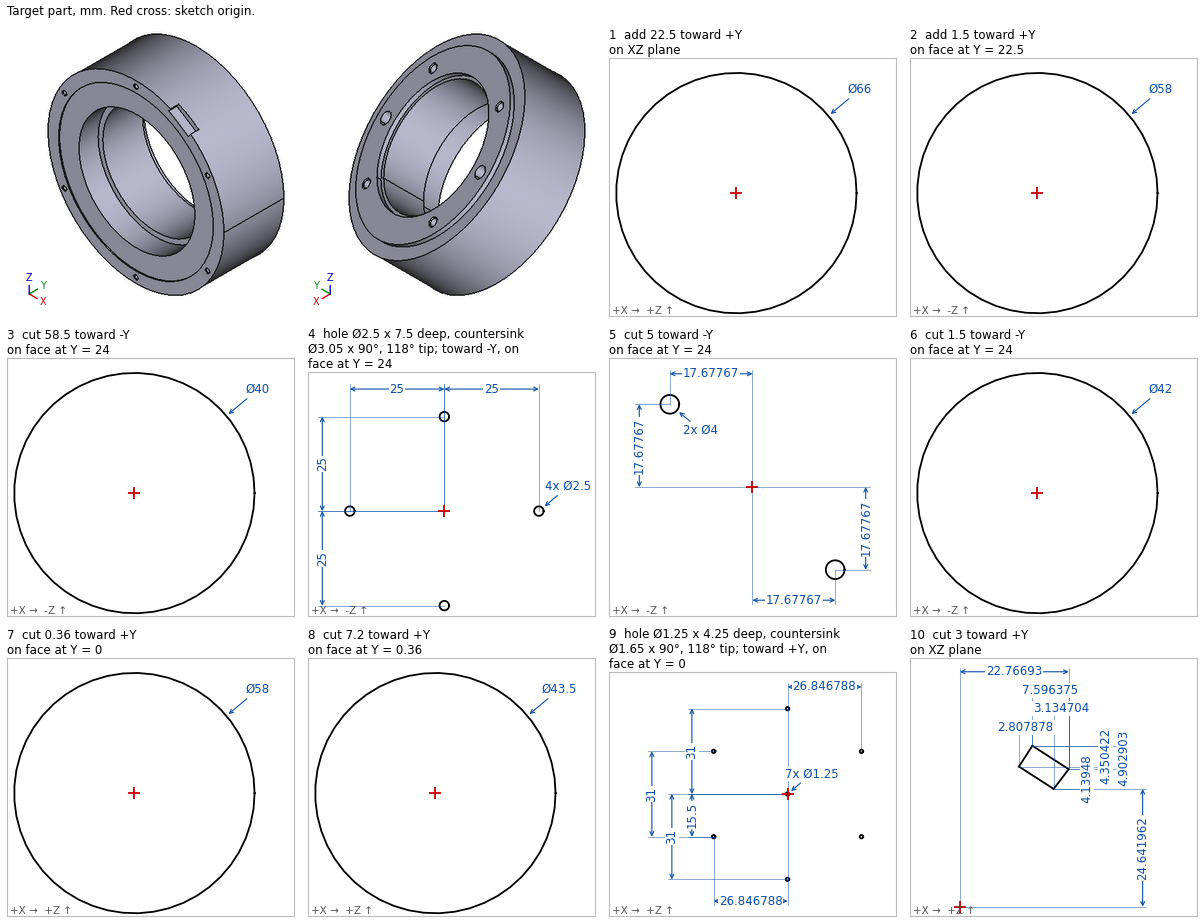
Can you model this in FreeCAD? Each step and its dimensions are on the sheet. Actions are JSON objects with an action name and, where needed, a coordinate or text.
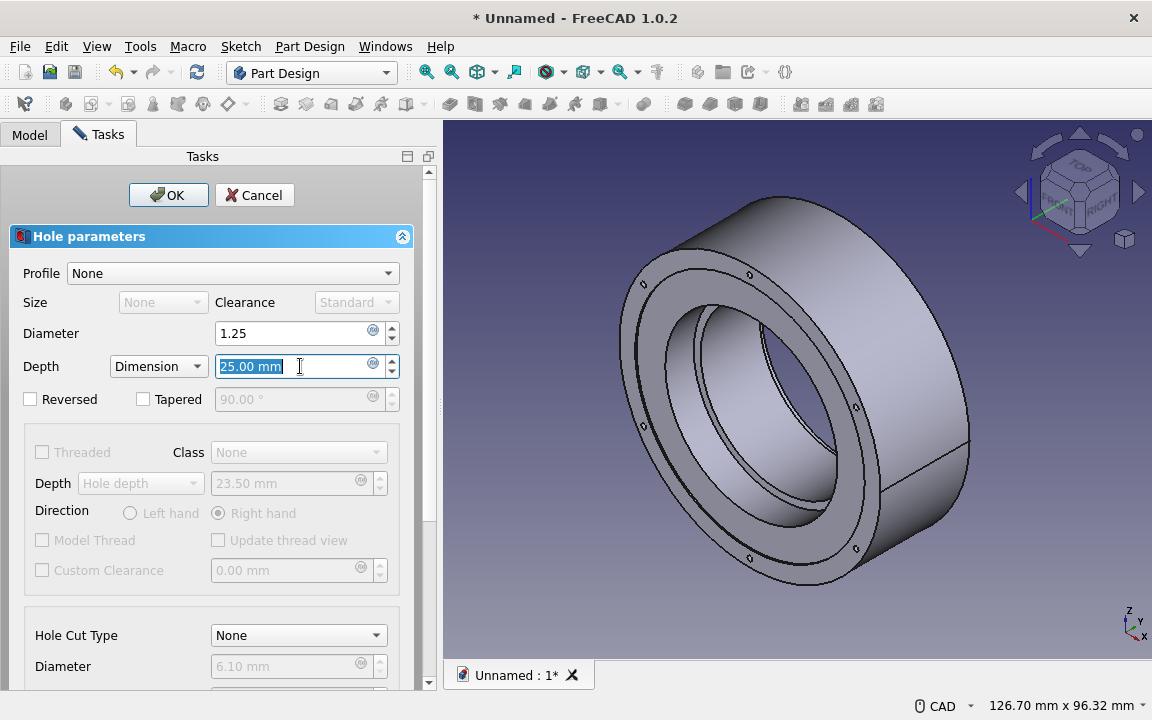
{"action": "type", "text": "4.25"}
{"action": "key", "text": "Tab"}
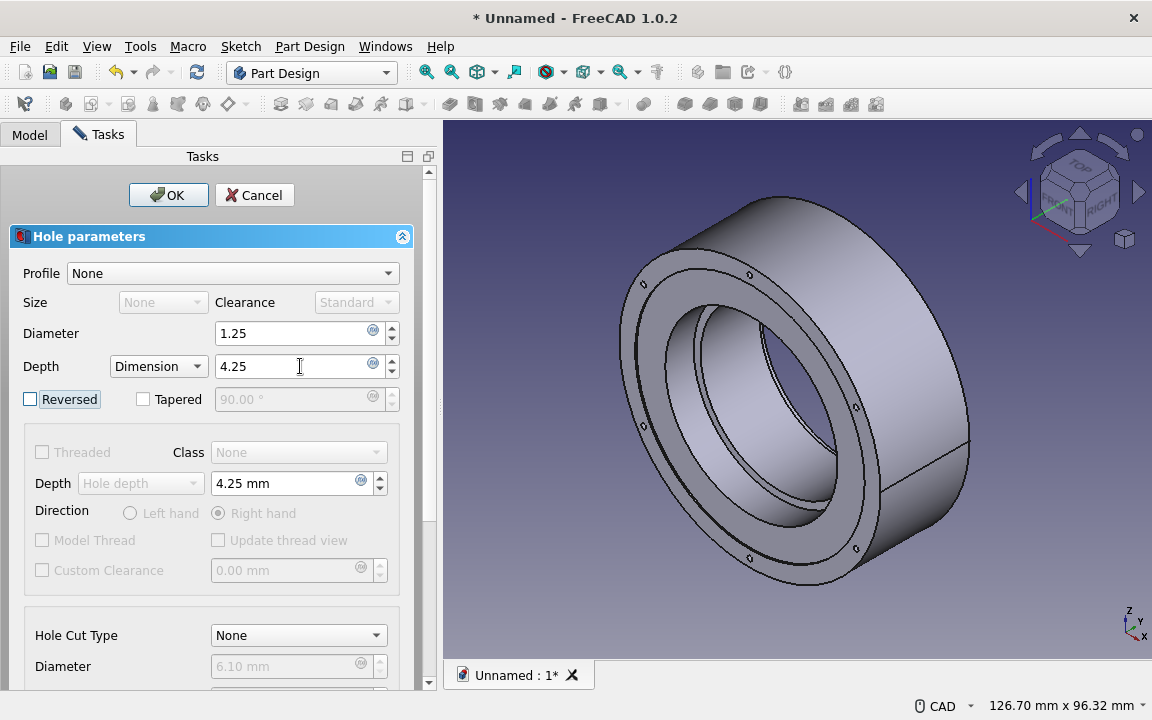
{"action": "left_click", "coordinate": [300, 636]}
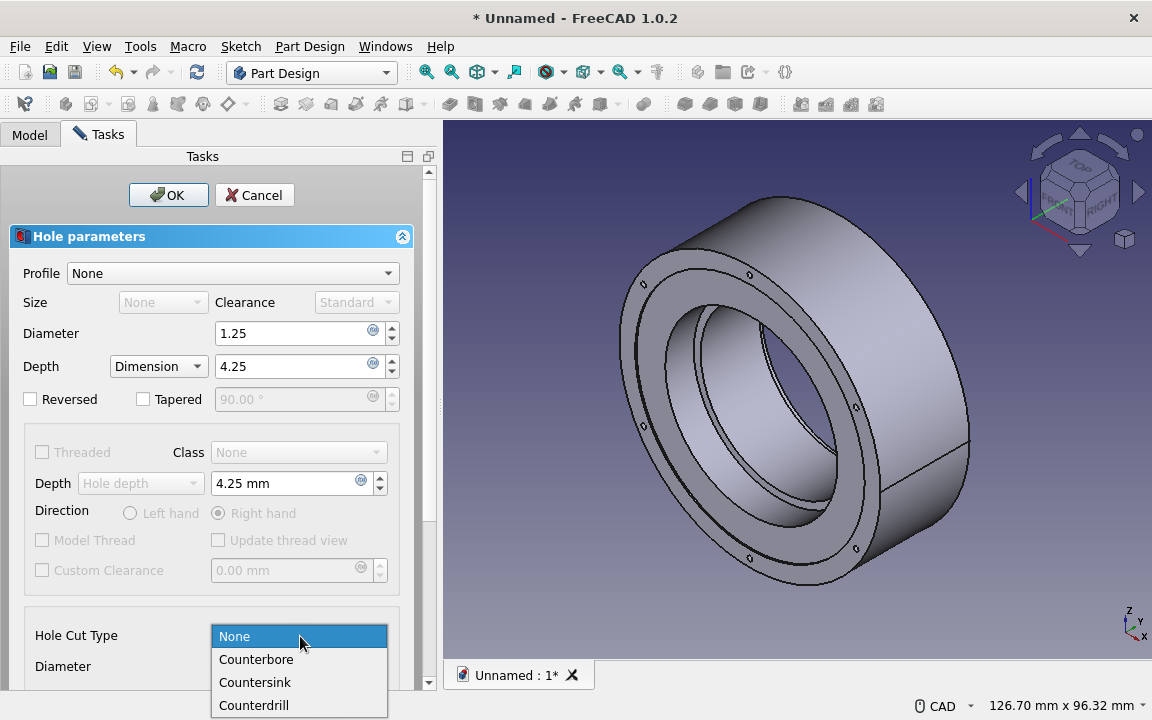
{"action": "left_click", "coordinate": [298, 682]}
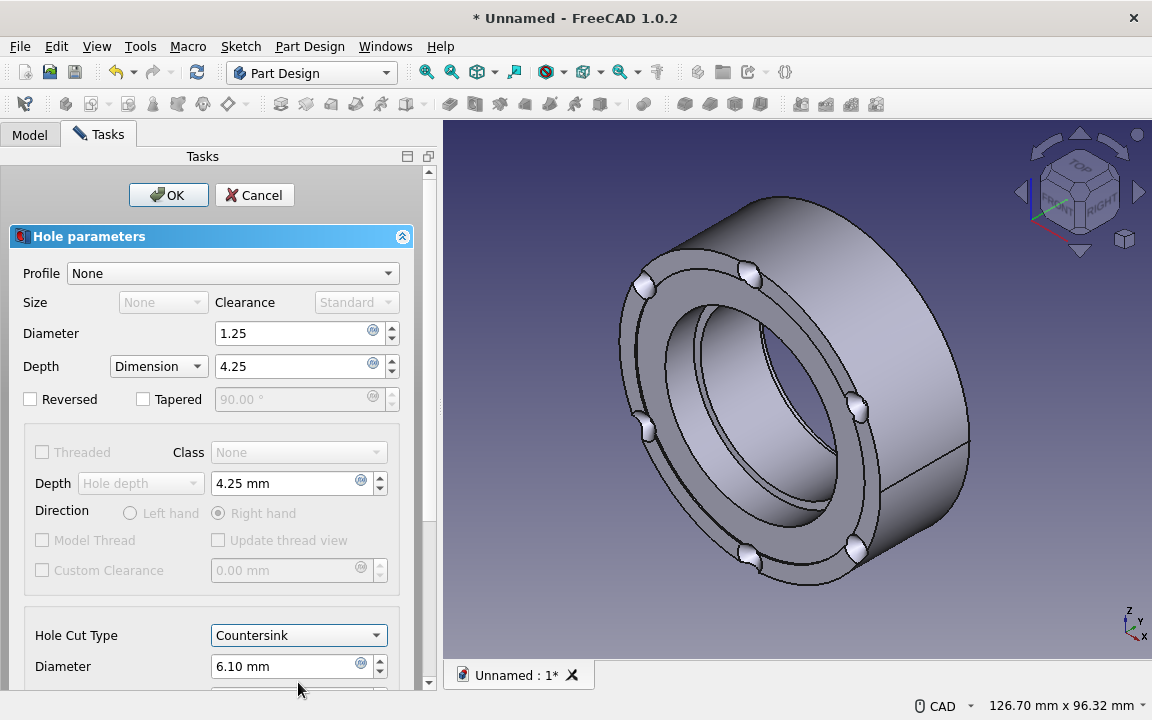
{"action": "triple_click", "coordinate": [292, 666]}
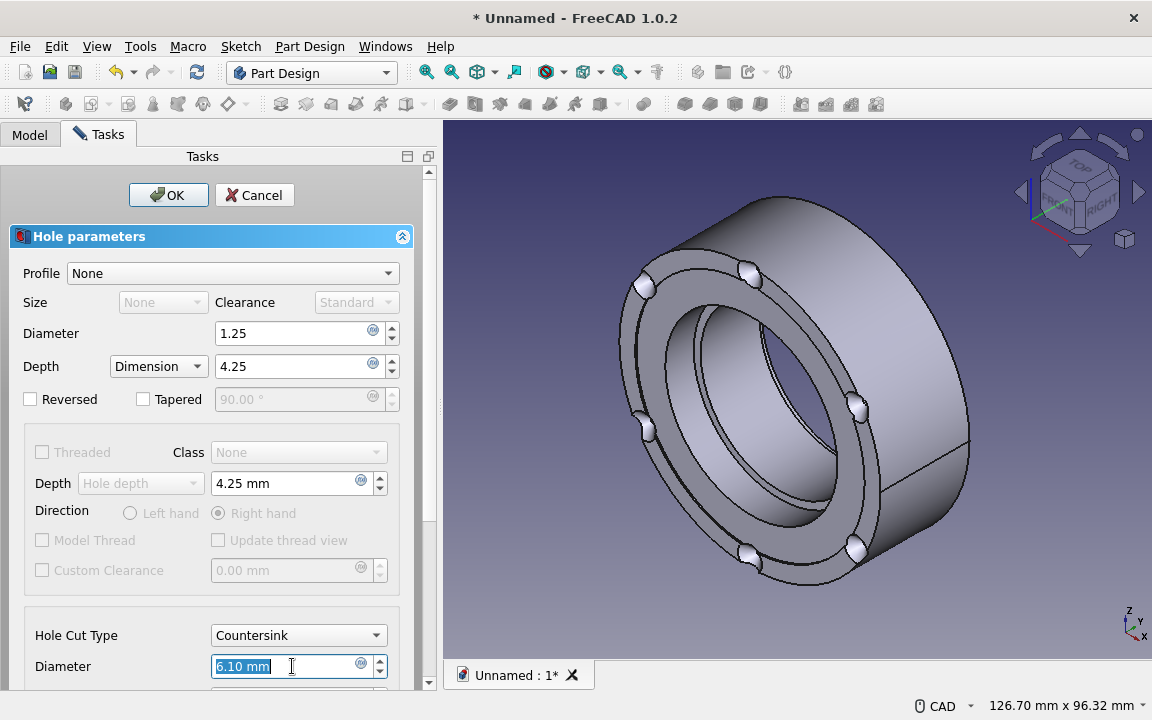
{"action": "type", "text": "1.65"}
{"action": "key", "text": "Tab"}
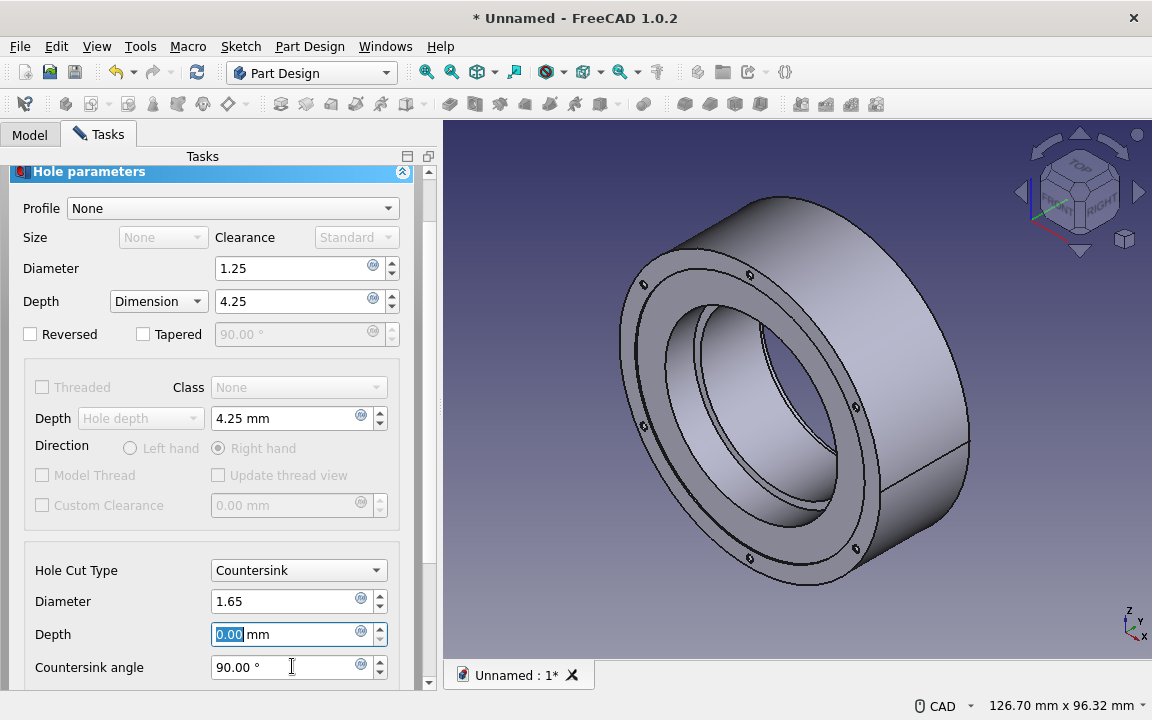
{"action": "scroll", "coordinate": [429, 428], "scroll_direction": "up", "scroll_amount": 2}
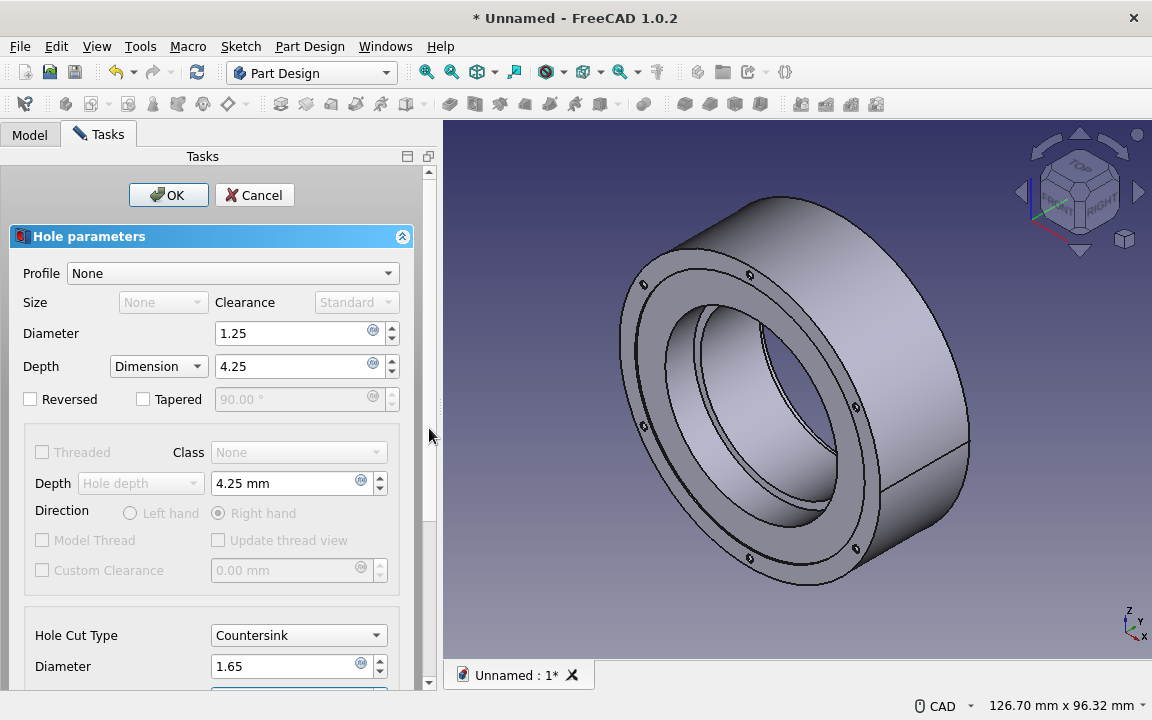
{"action": "left_click", "coordinate": [169, 195]}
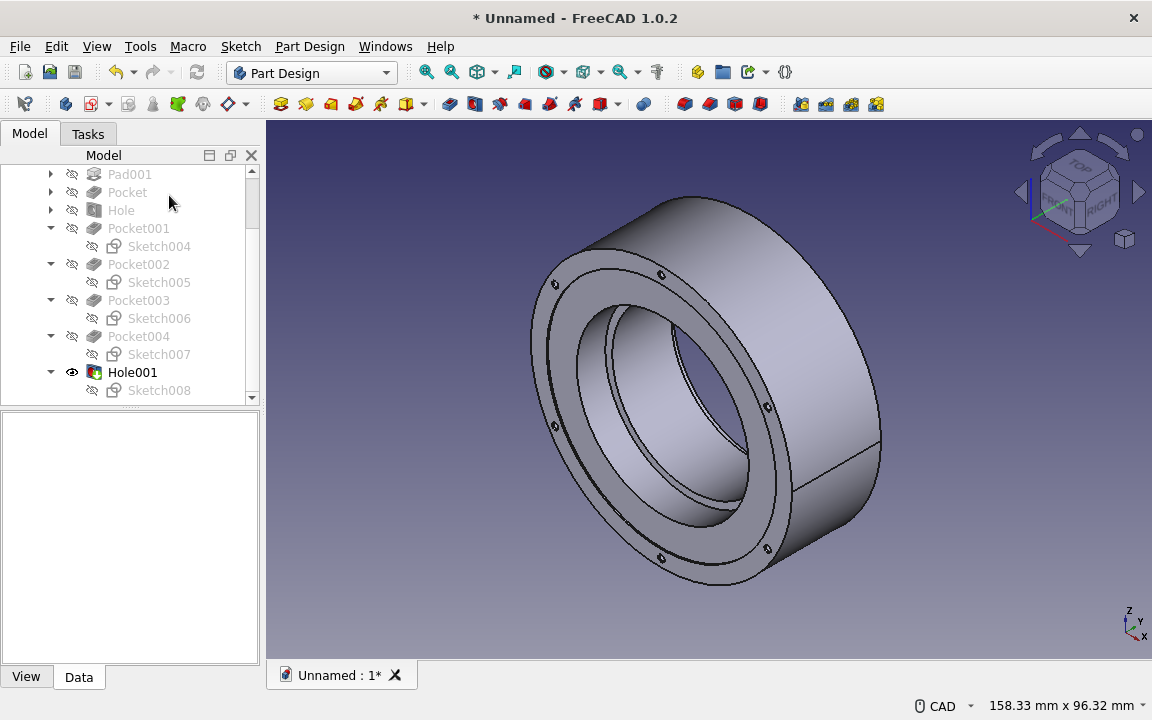
{"action": "left_click", "coordinate": [90, 104]}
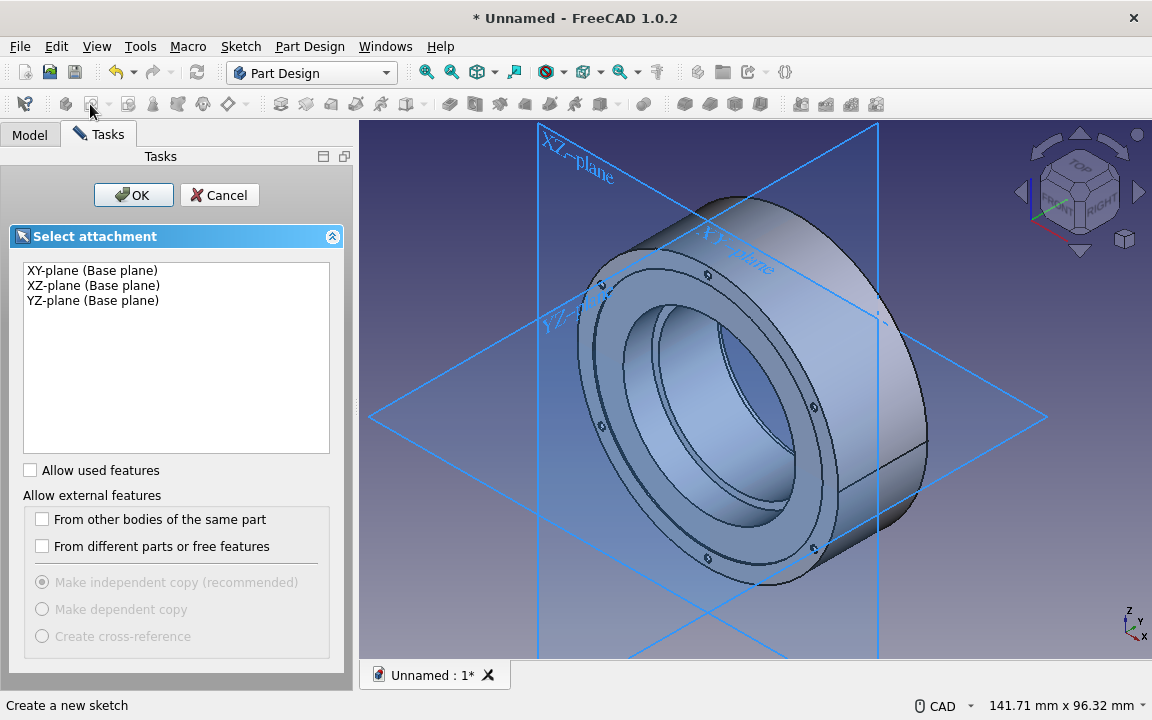
{"action": "left_click", "coordinate": [84, 286]}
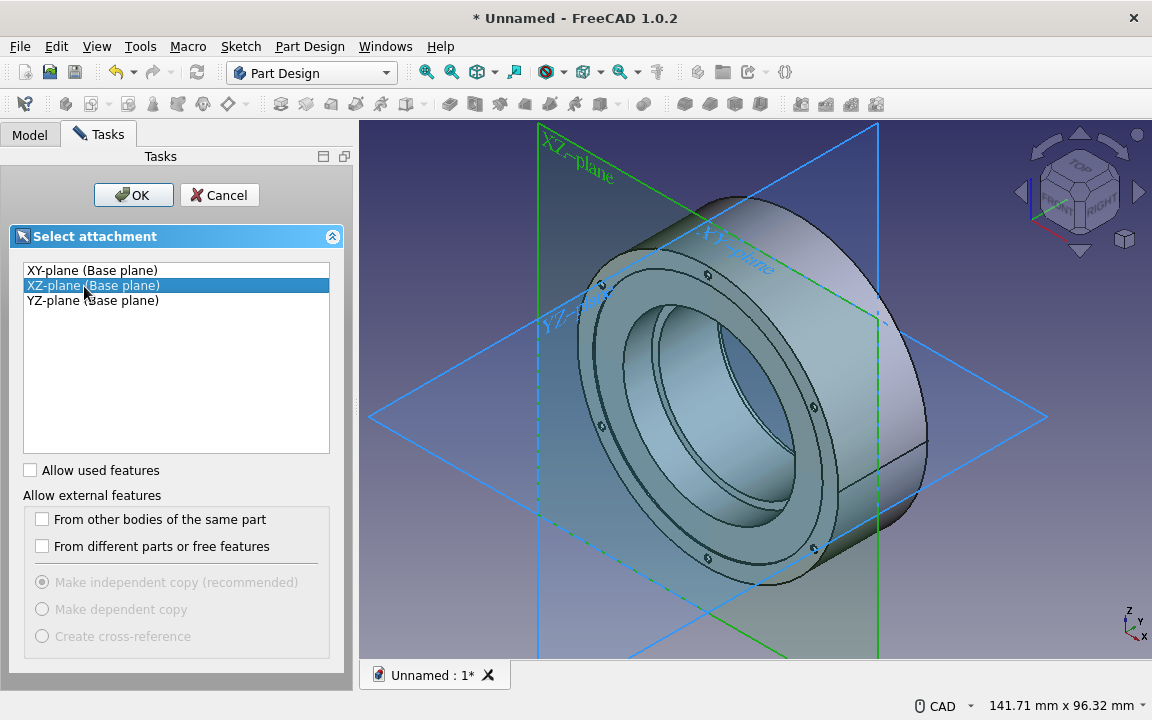
{"action": "left_click", "coordinate": [134, 195]}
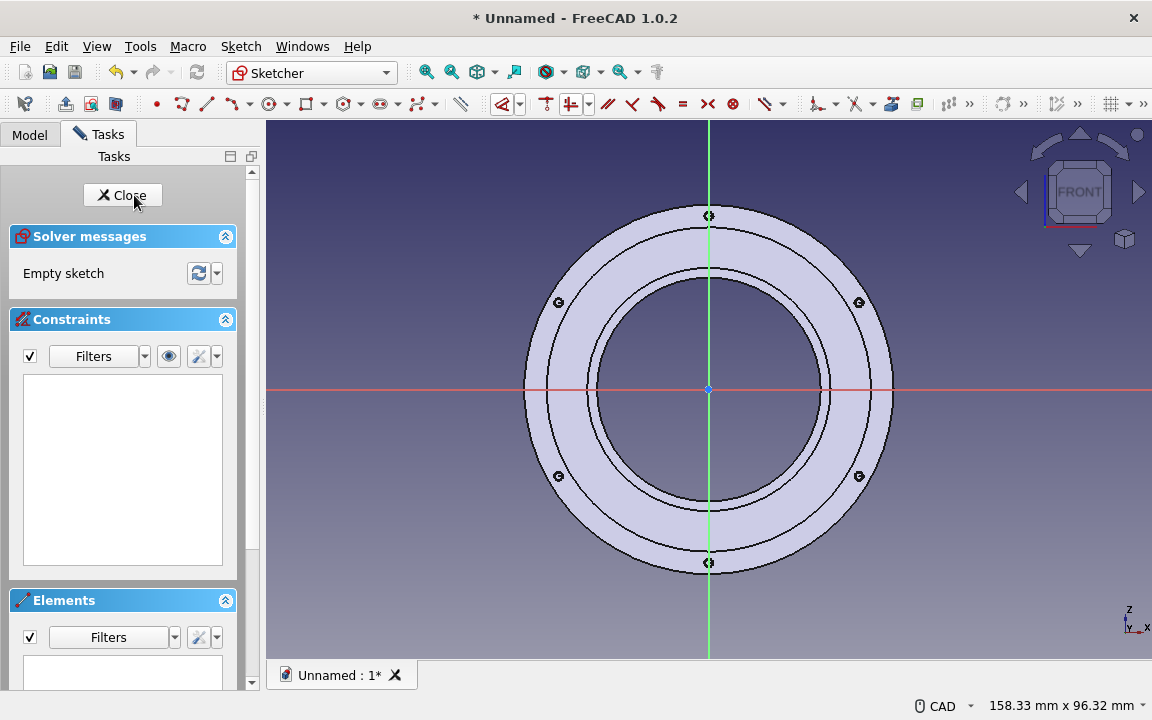
{"action": "scroll", "coordinate": [833, 201], "scroll_direction": "up", "scroll_amount": 10}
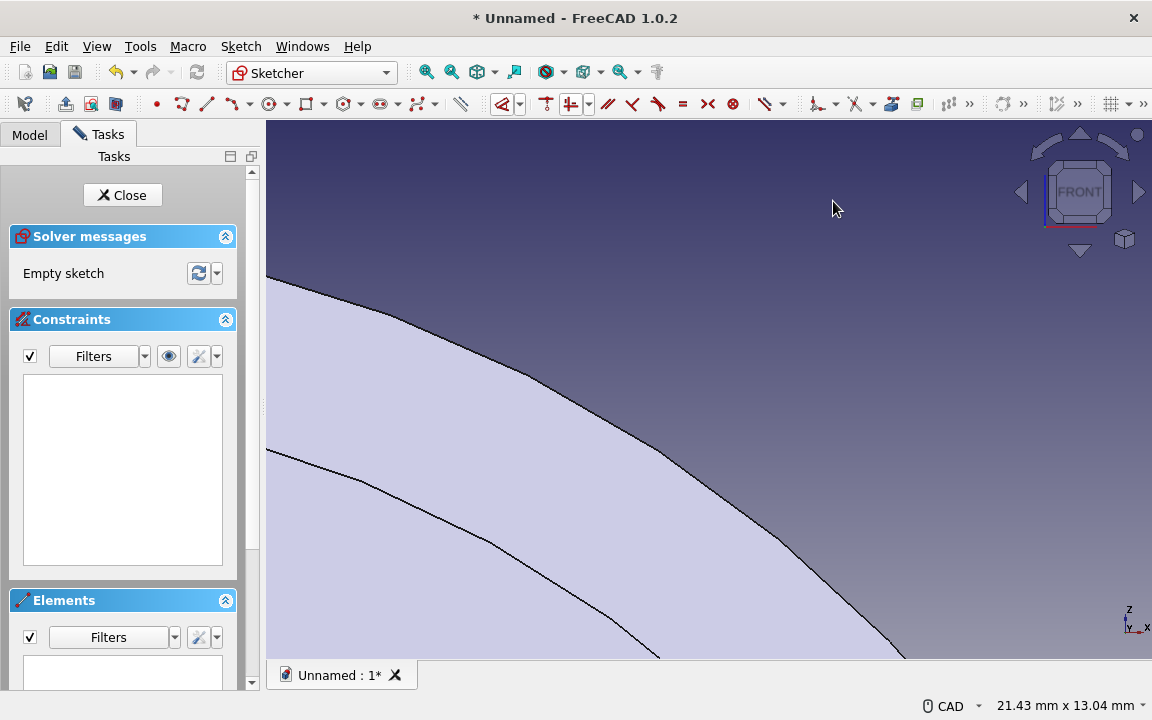
{"action": "left_click", "coordinate": [182, 104]}